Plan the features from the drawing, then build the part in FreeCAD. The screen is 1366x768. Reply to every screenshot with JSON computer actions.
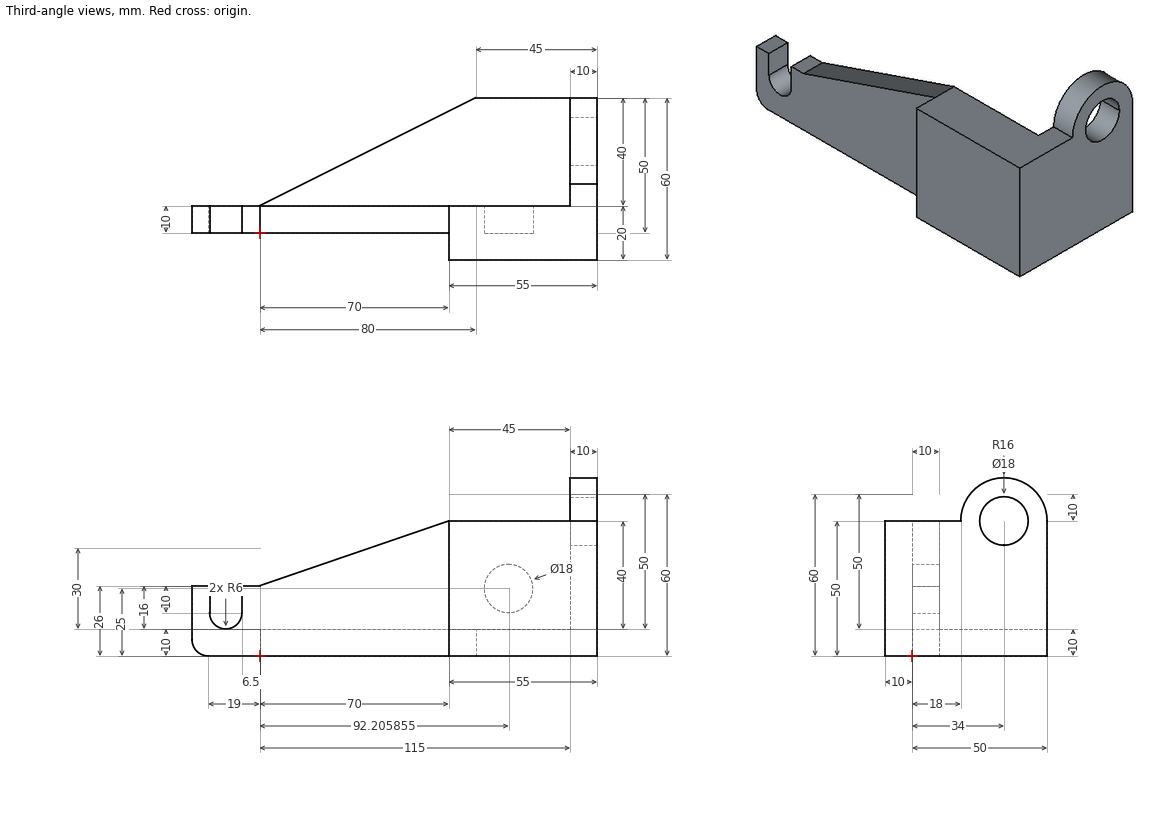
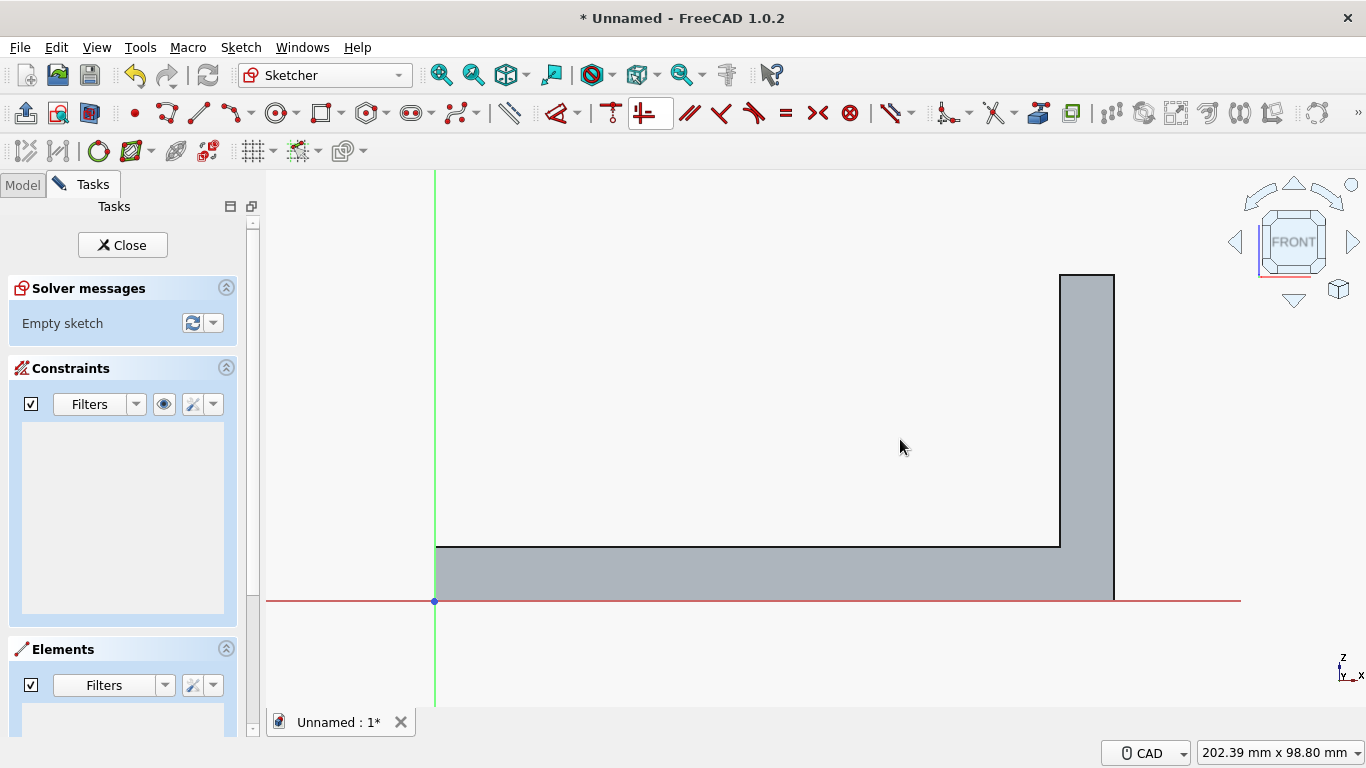
{"action": "left_click", "coordinate": [168, 114]}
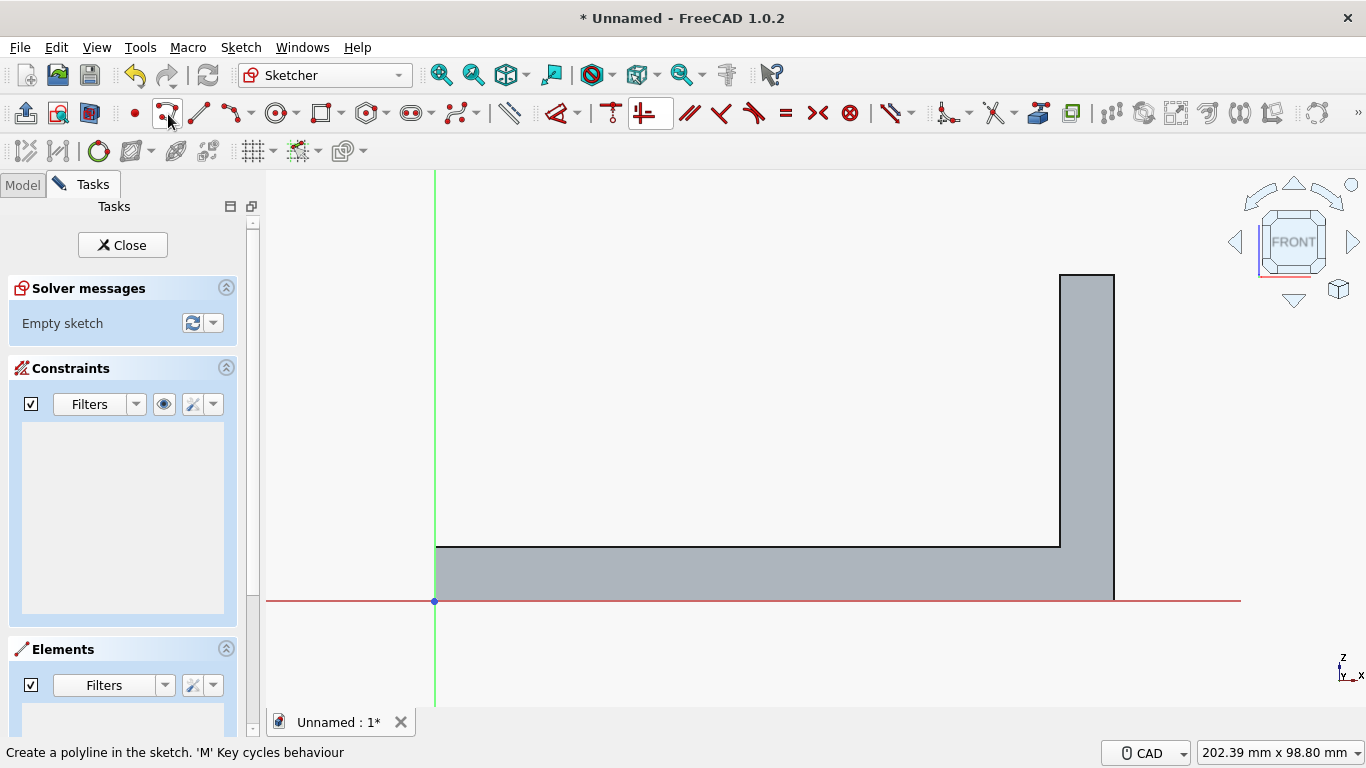
{"action": "left_click", "coordinate": [435, 547]}
{"action": "left_click", "coordinate": [1060, 547]}
{"action": "left_click", "coordinate": [1060, 275]}
{"action": "left_click", "coordinate": [815, 275]}
{"action": "left_click", "coordinate": [444, 384]}
{"action": "left_click", "coordinate": [435, 548]}
{"action": "key", "text": "Escape"}
{"action": "key", "text": "Escape"}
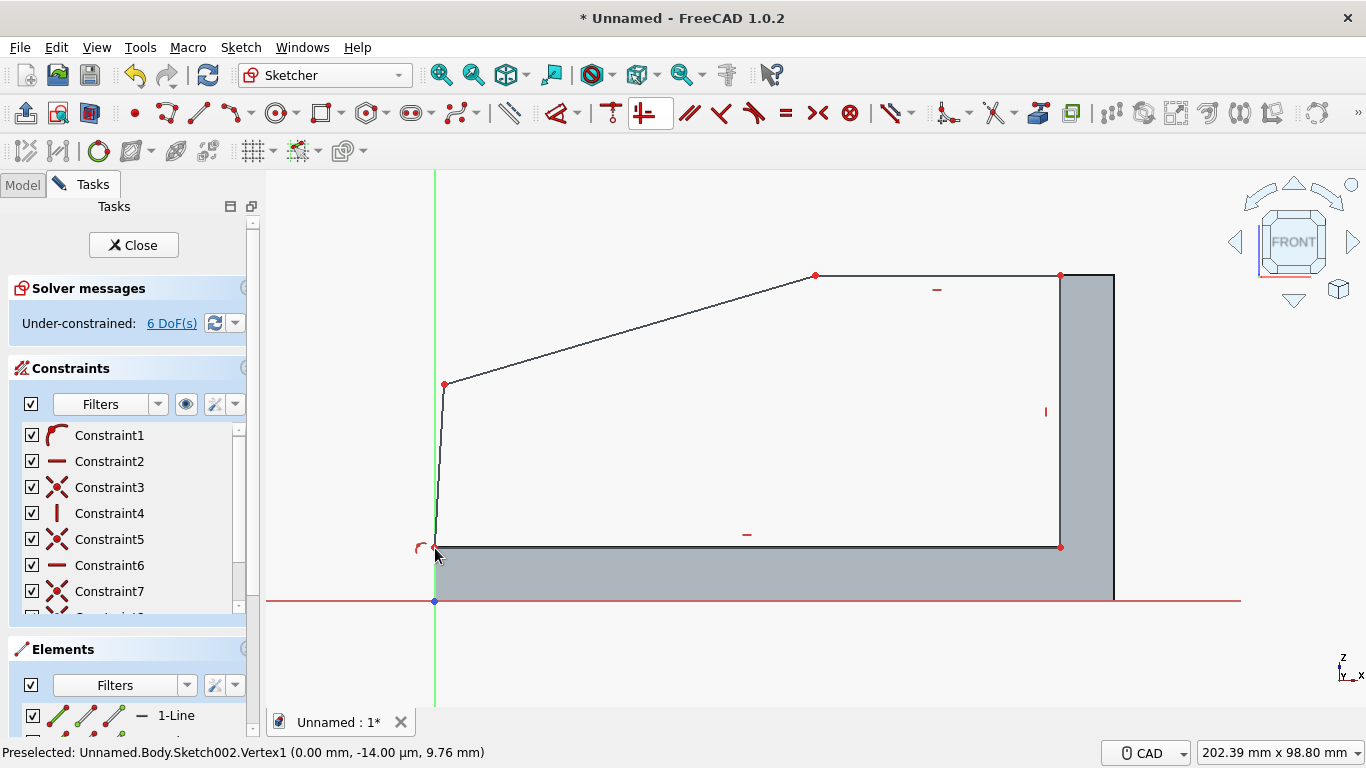
{"action": "left_click", "coordinate": [437, 499]}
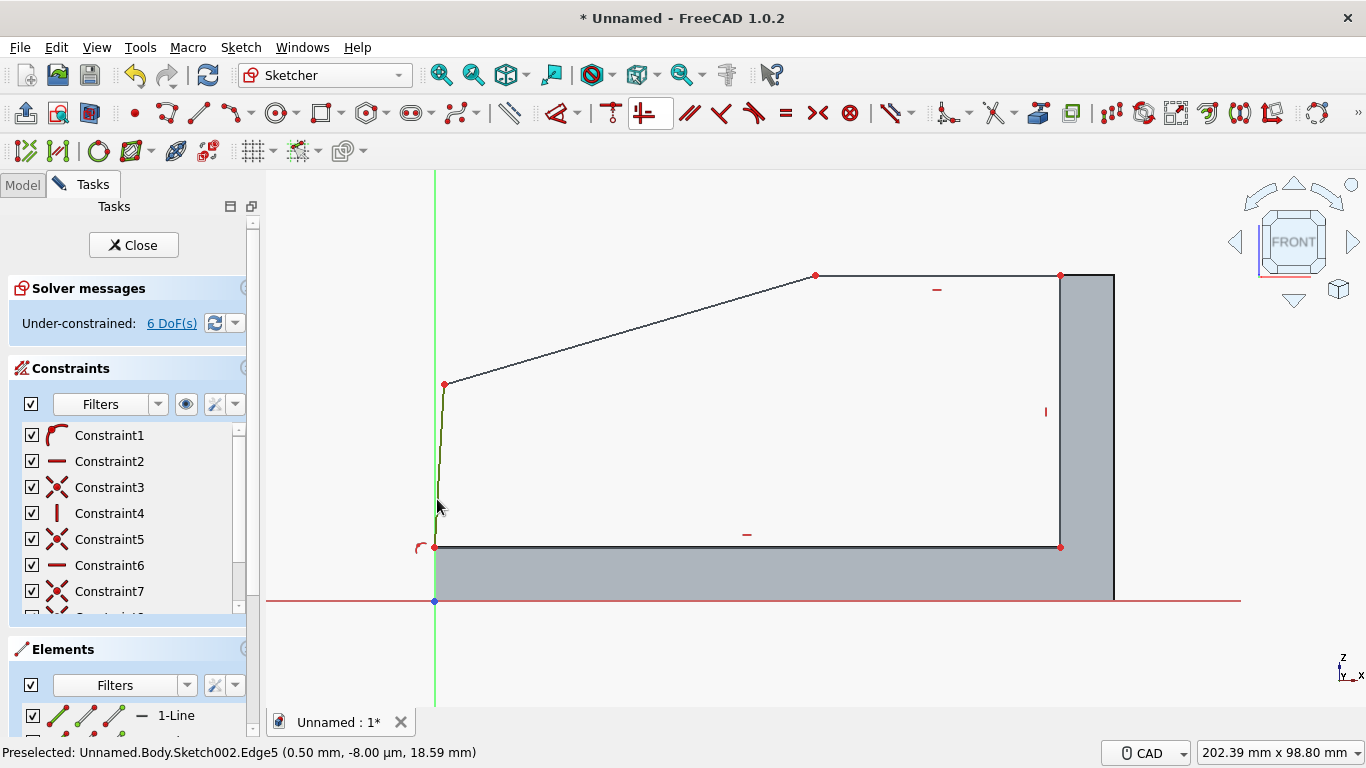
{"action": "key", "text": "v"}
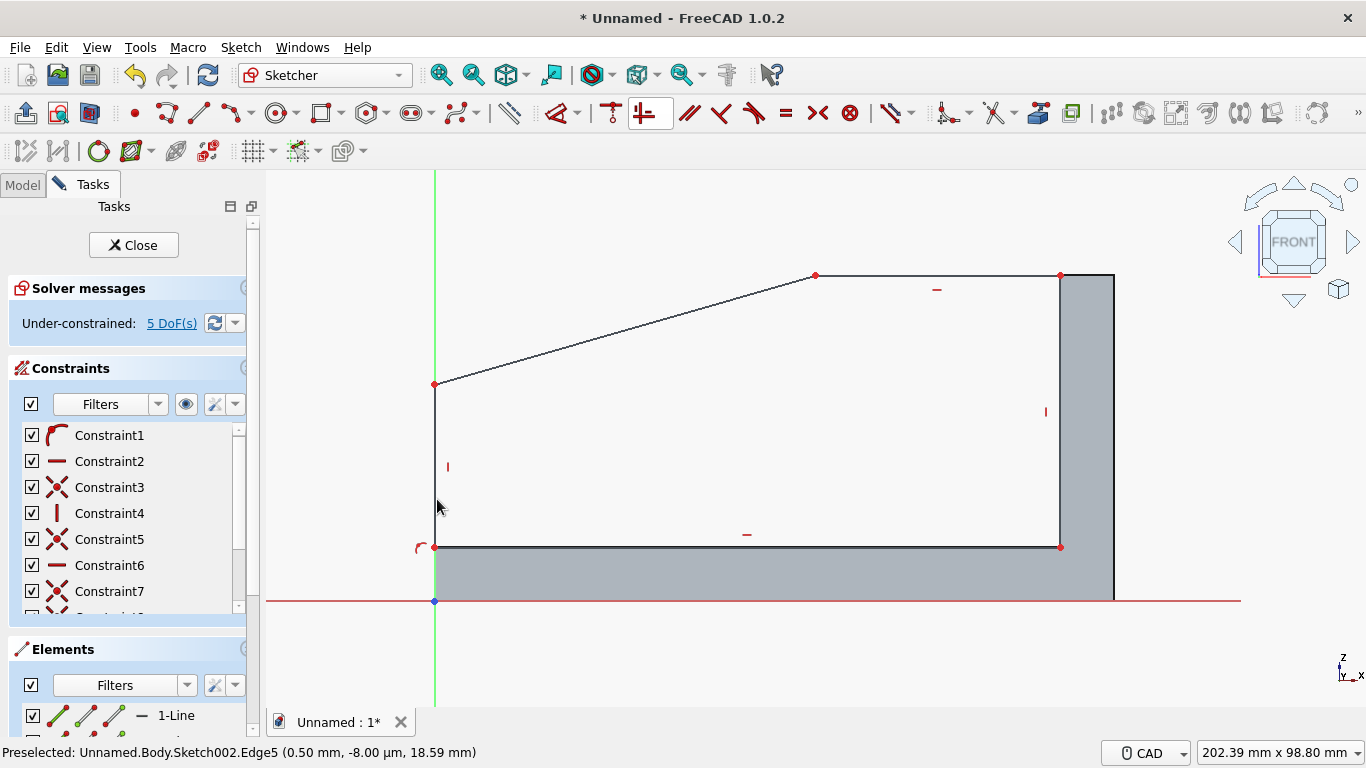
{"action": "left_click", "coordinate": [556, 114]}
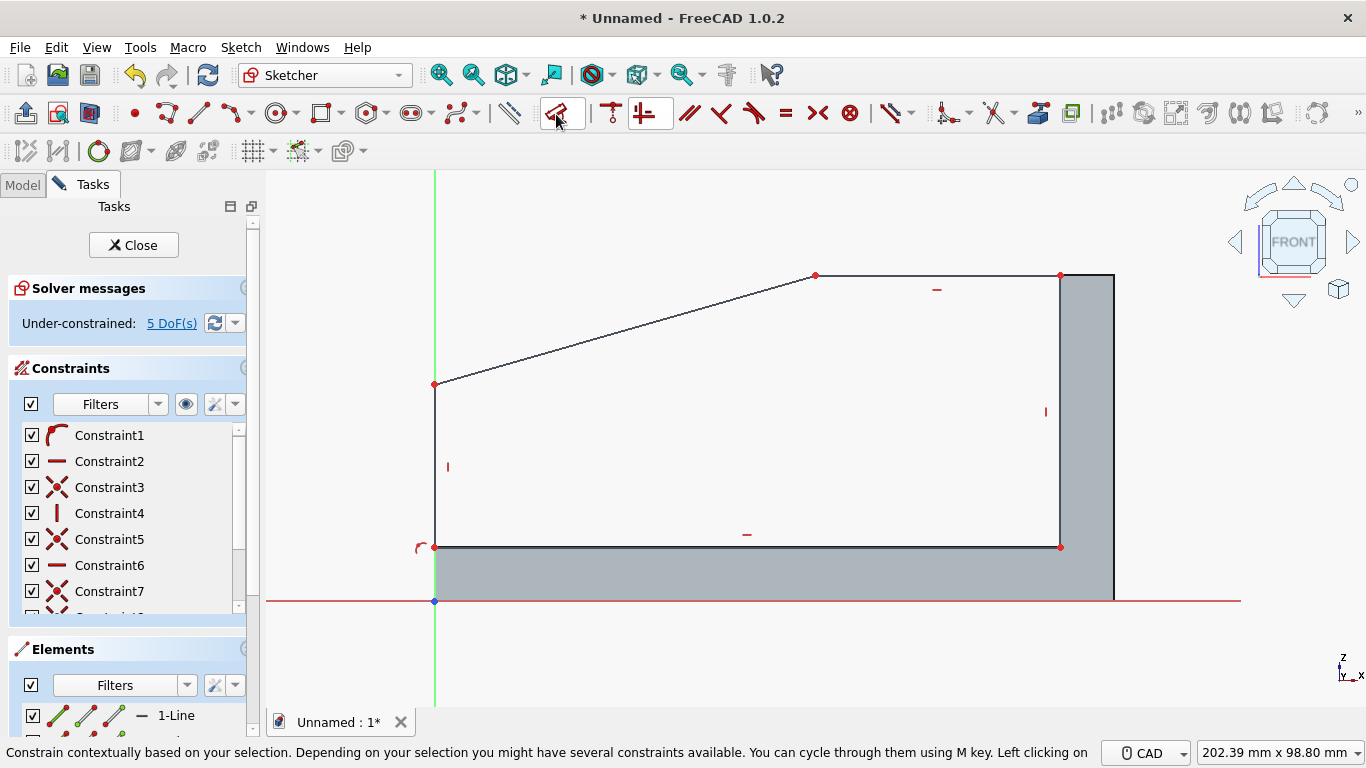
{"action": "left_click", "coordinate": [1060, 466]}
{"action": "left_click", "coordinate": [1094, 412]}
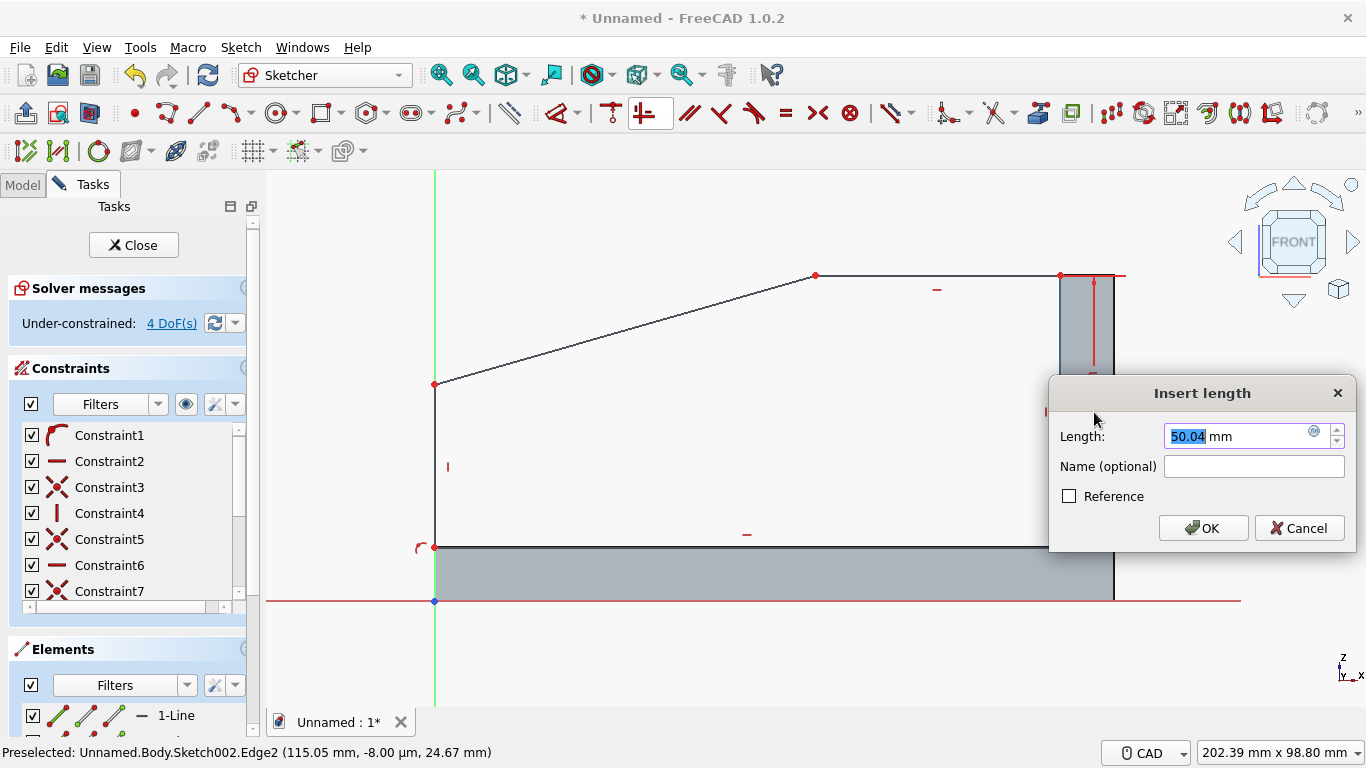
{"action": "type", "text": "50"}
{"action": "key", "text": "Return"}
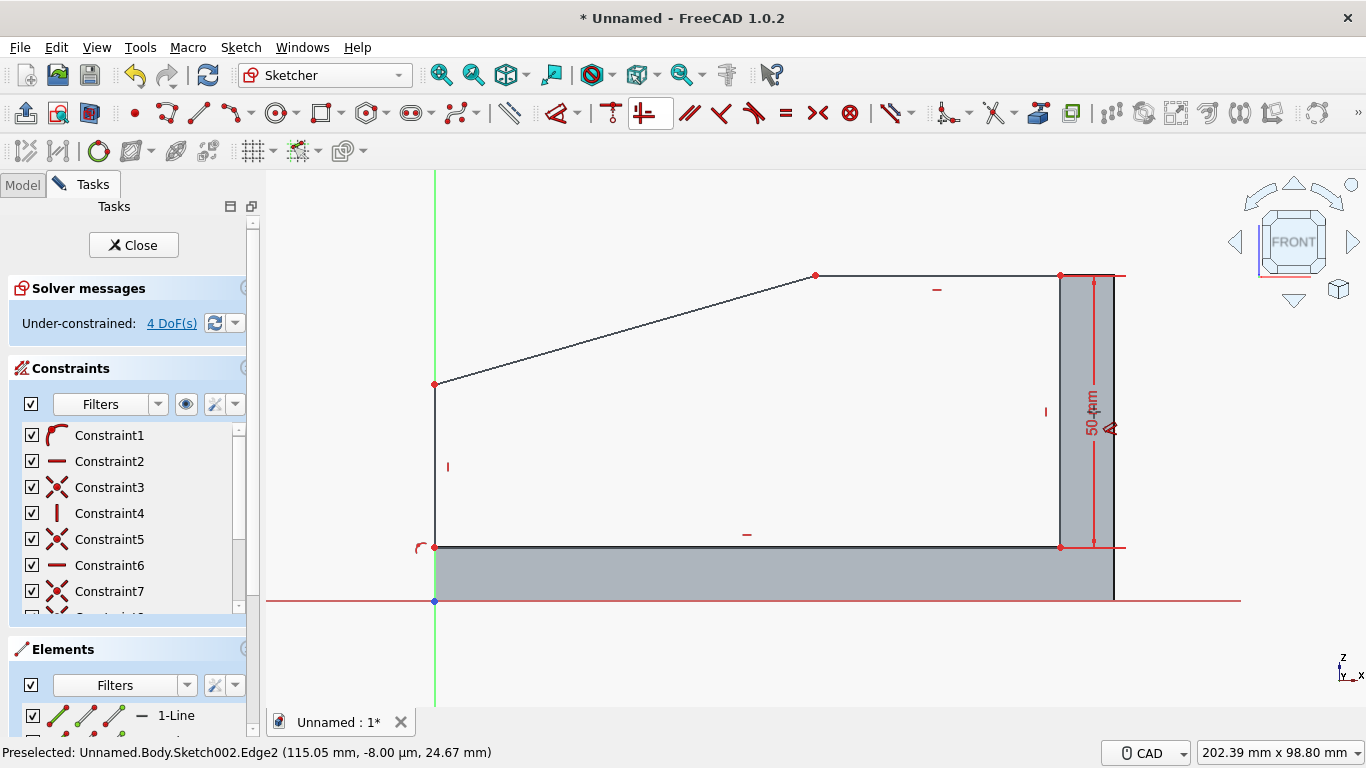
{"action": "left_click", "coordinate": [987, 276]}
{"action": "left_click", "coordinate": [938, 242]}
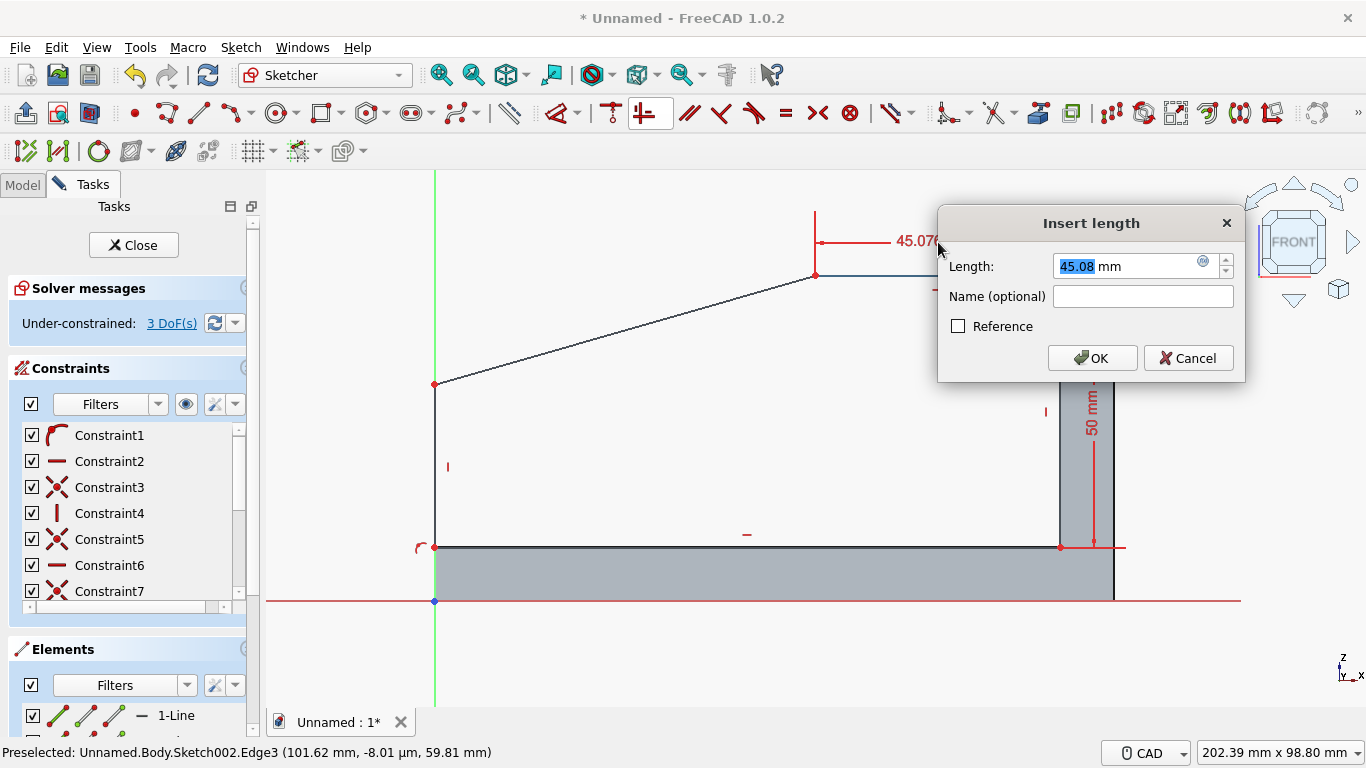
{"action": "type", "text": "45"}
{"action": "key", "text": "Return"}